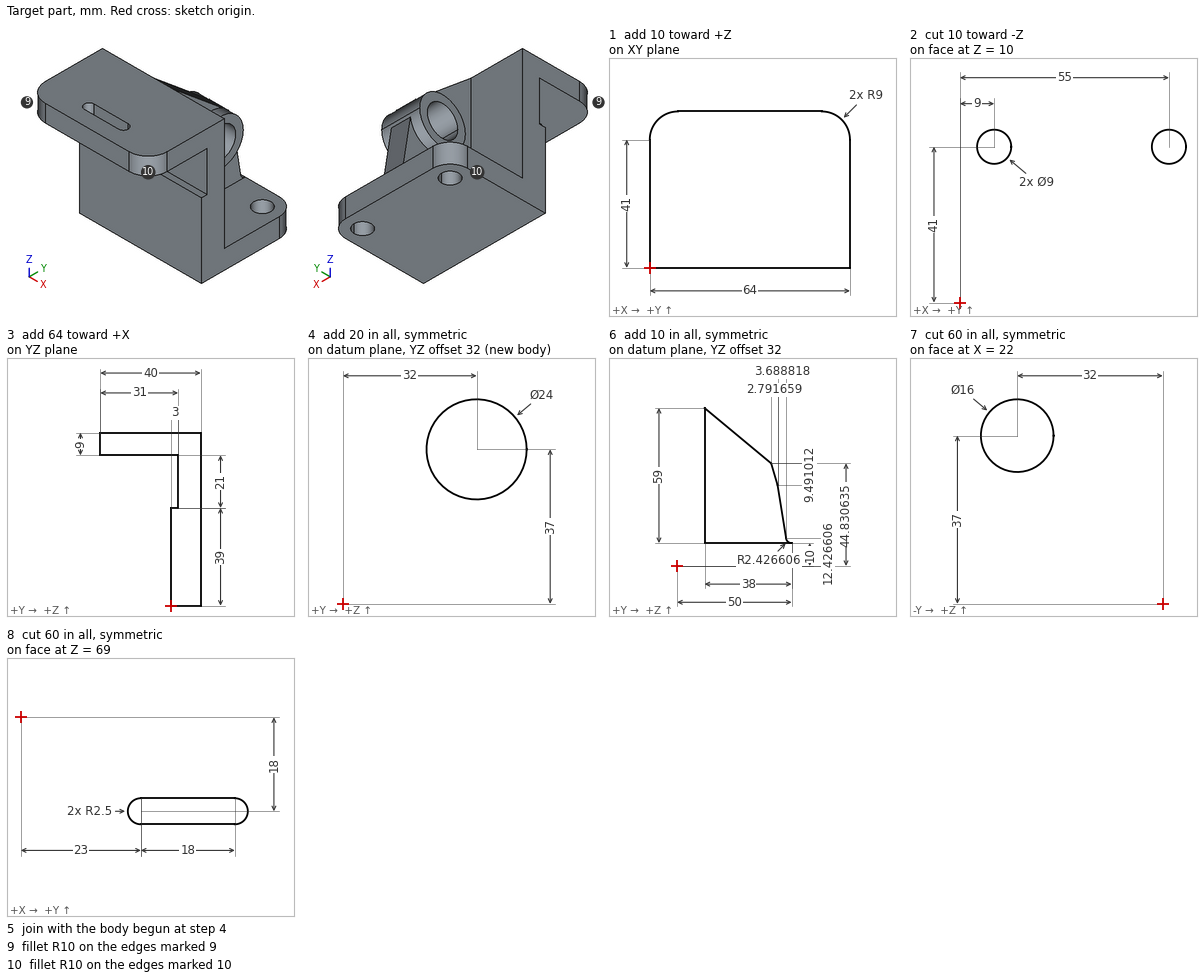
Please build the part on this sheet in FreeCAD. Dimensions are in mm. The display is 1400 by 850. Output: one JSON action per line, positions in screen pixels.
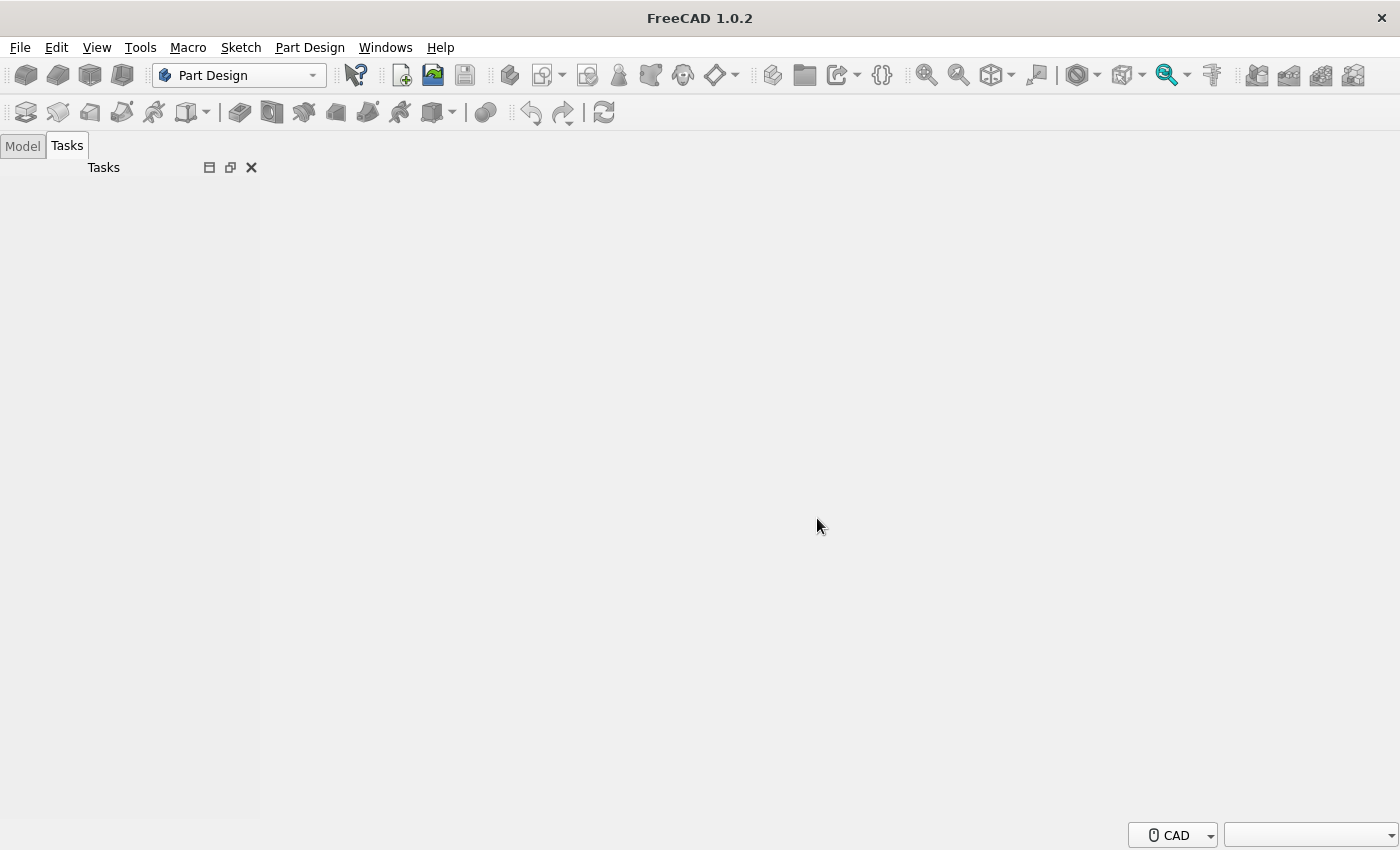
{"action": "left_click", "coordinate": [402, 76]}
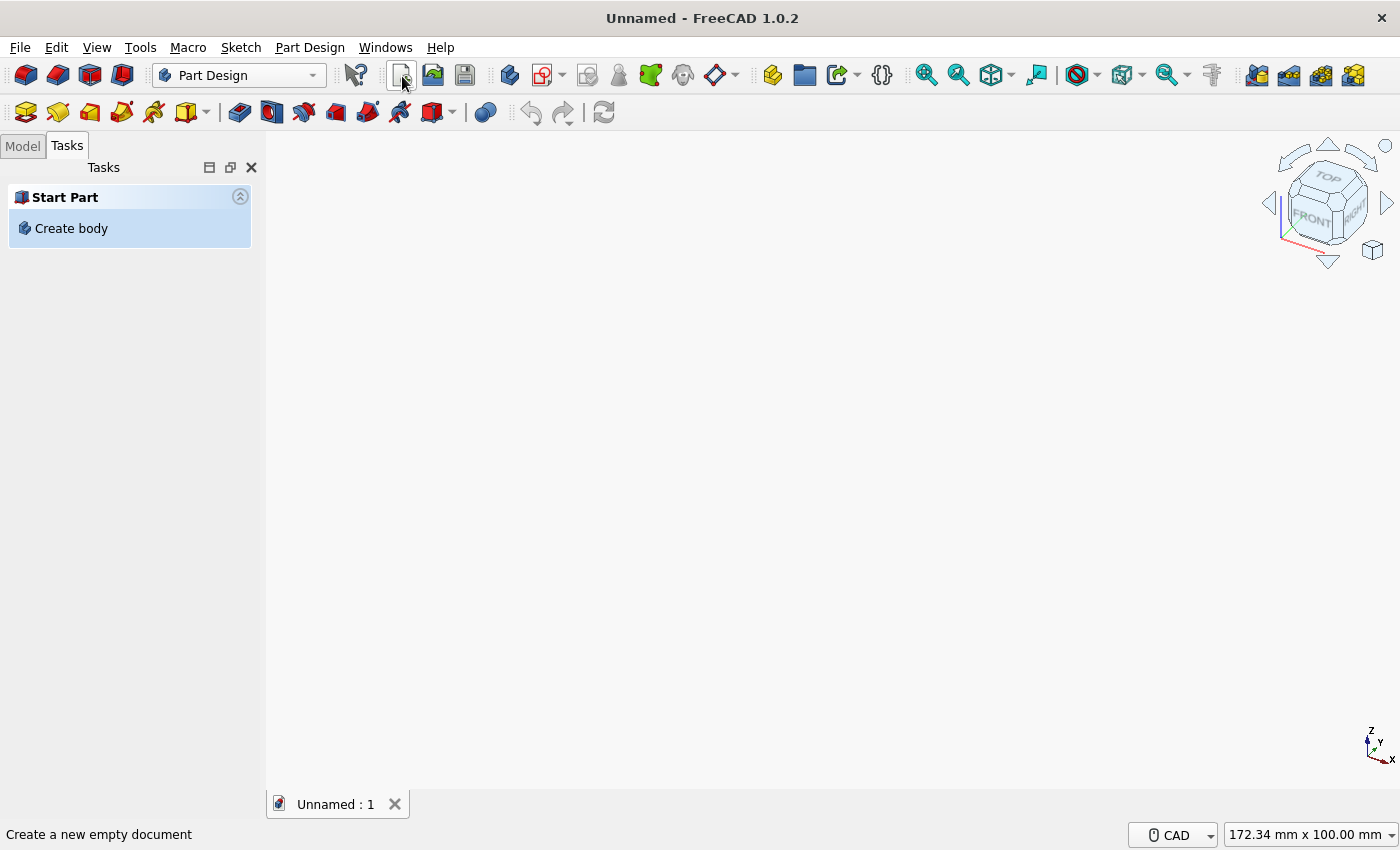
{"action": "left_click", "coordinate": [542, 76]}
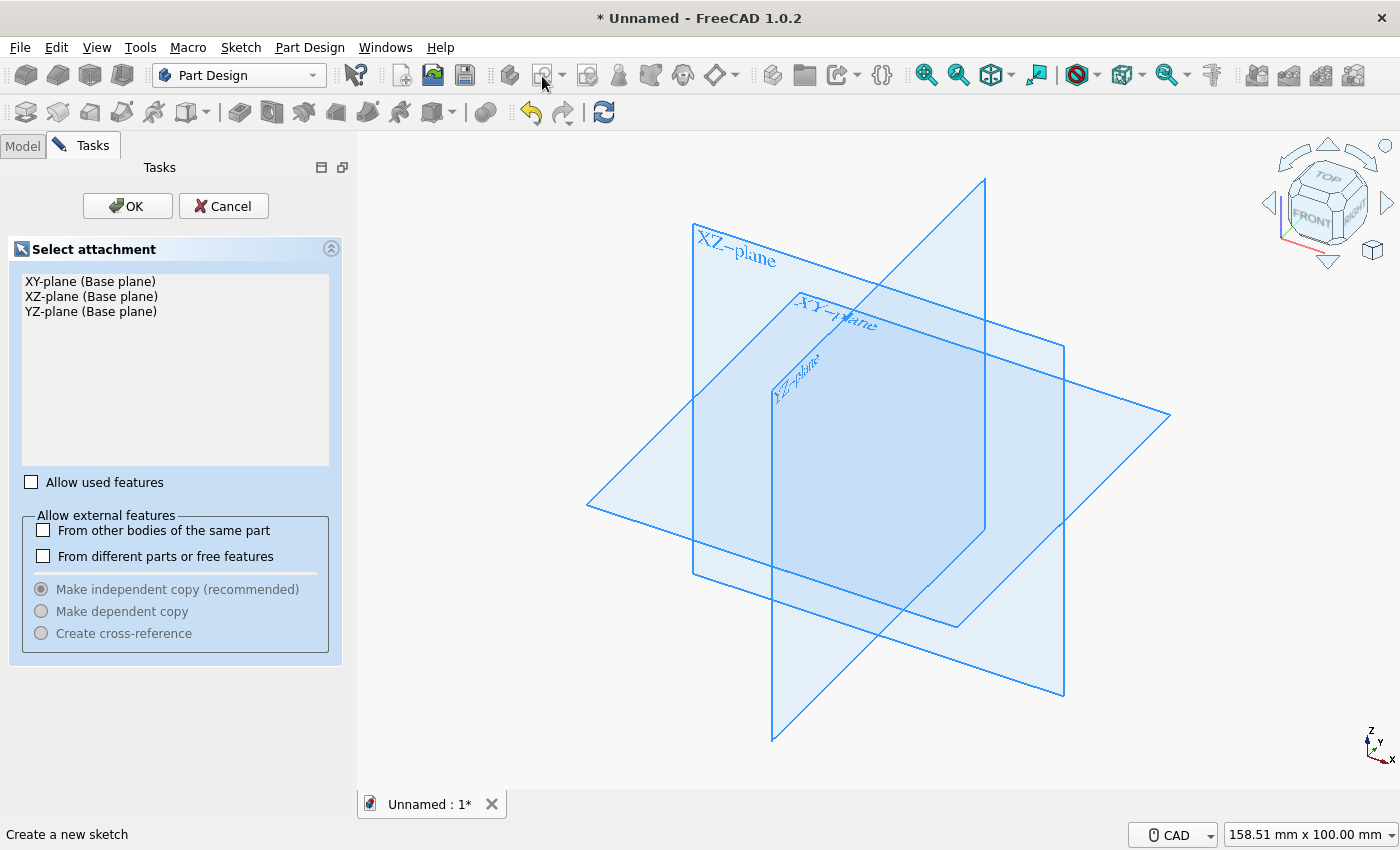
{"action": "left_click", "coordinate": [82, 282]}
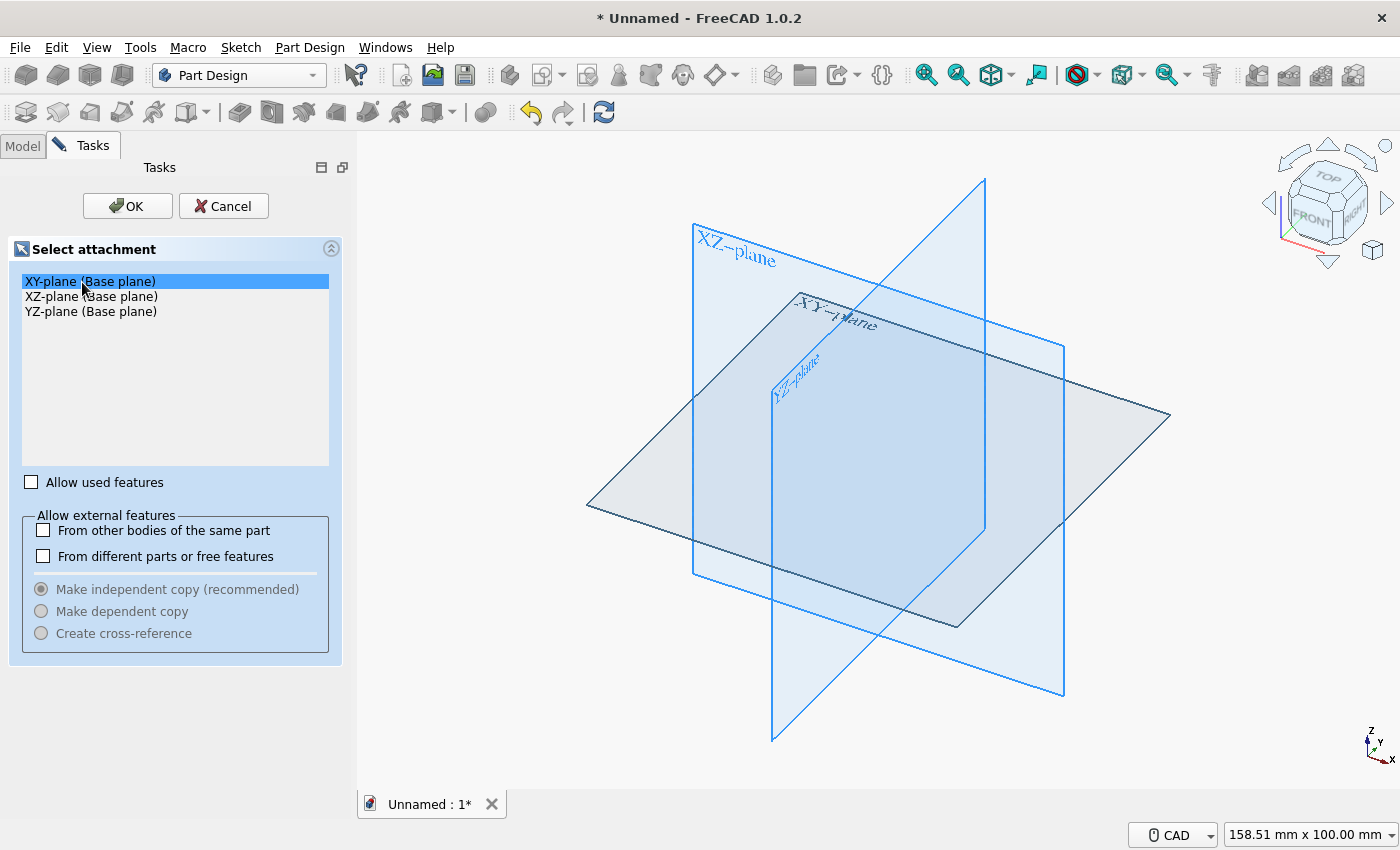
{"action": "left_click", "coordinate": [128, 206]}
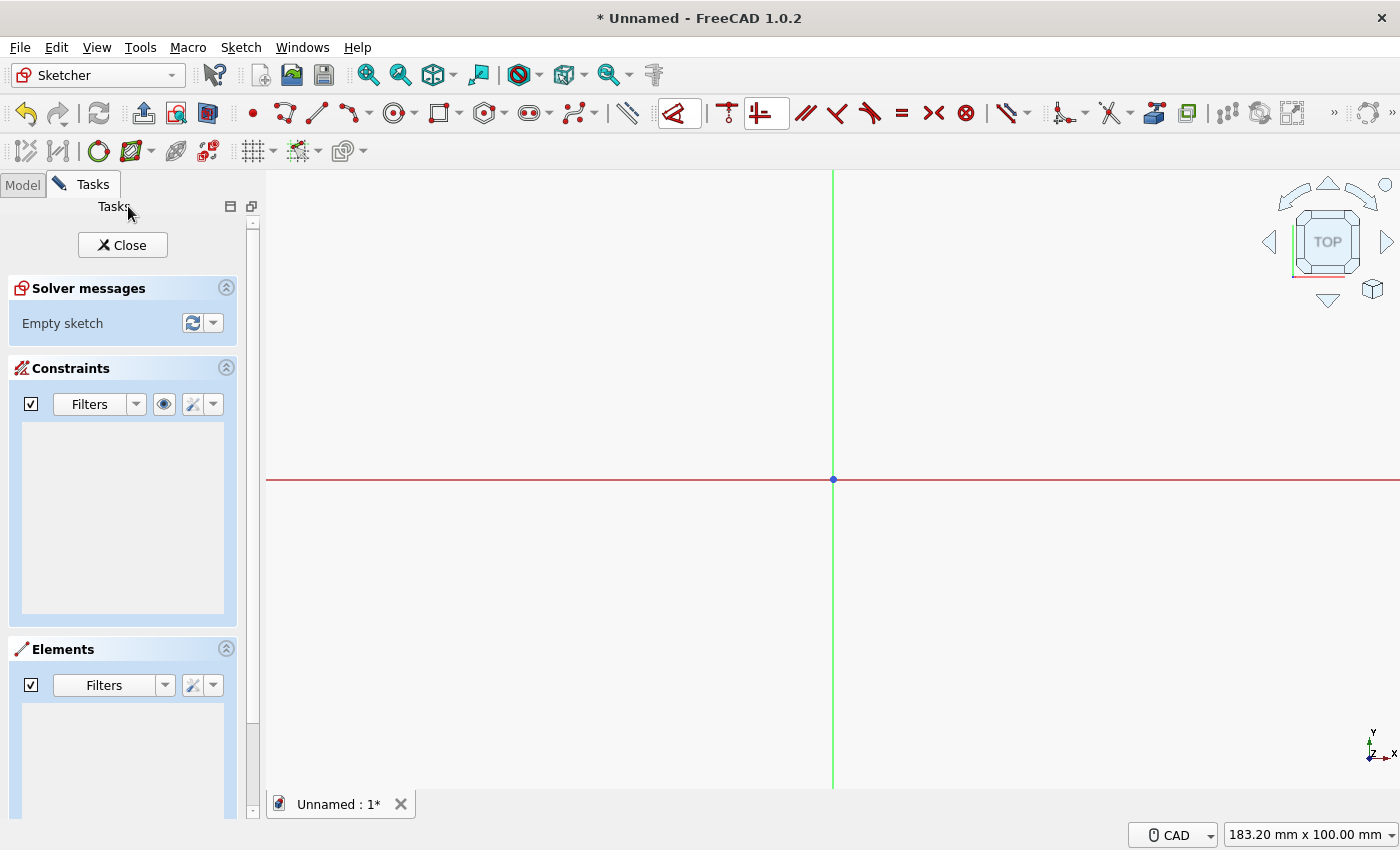
{"action": "scroll", "coordinate": [294, 761], "scroll_direction": "down", "scroll_amount": 1}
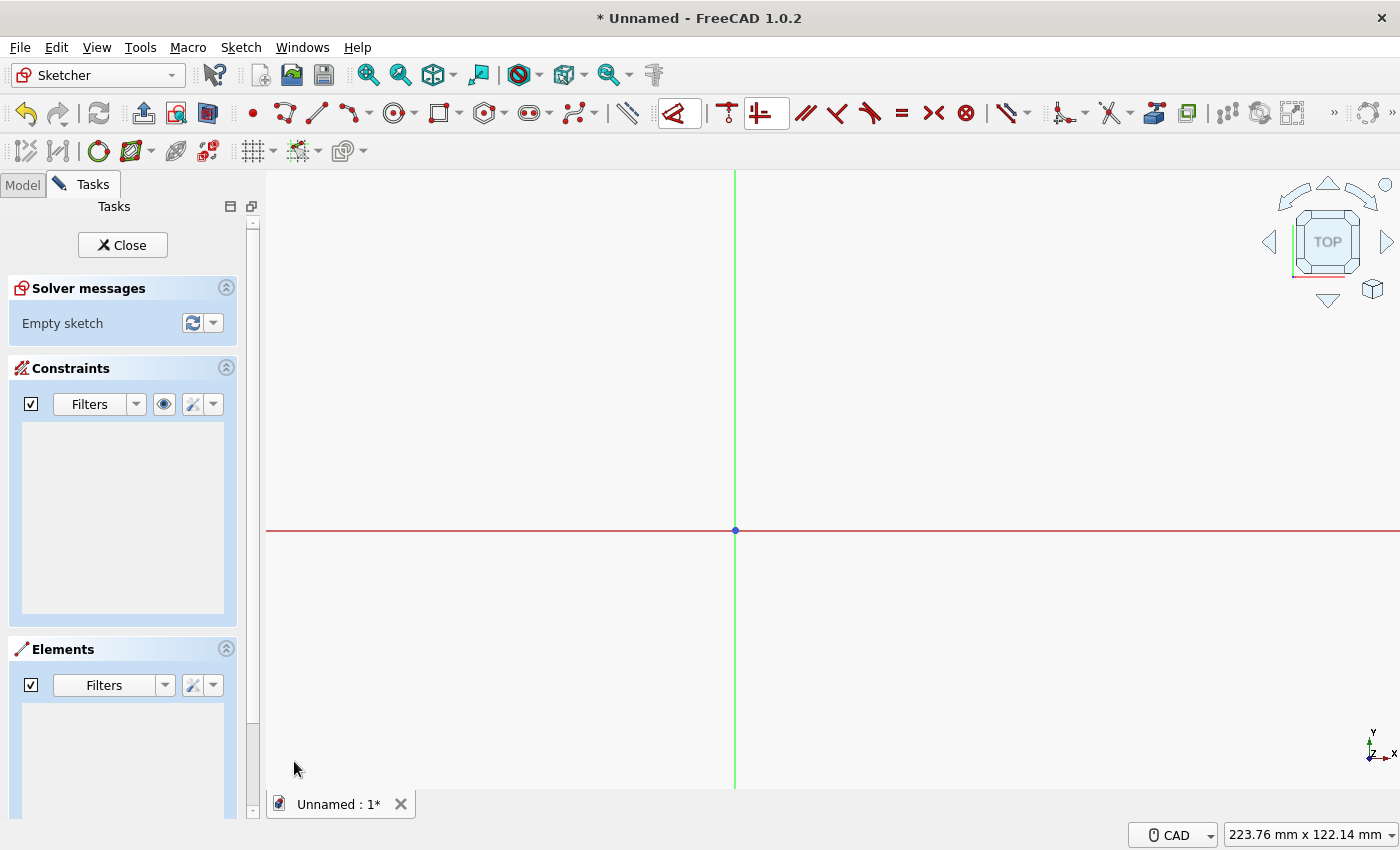
{"action": "scroll", "coordinate": [1168, 250], "scroll_direction": "up", "scroll_amount": 2}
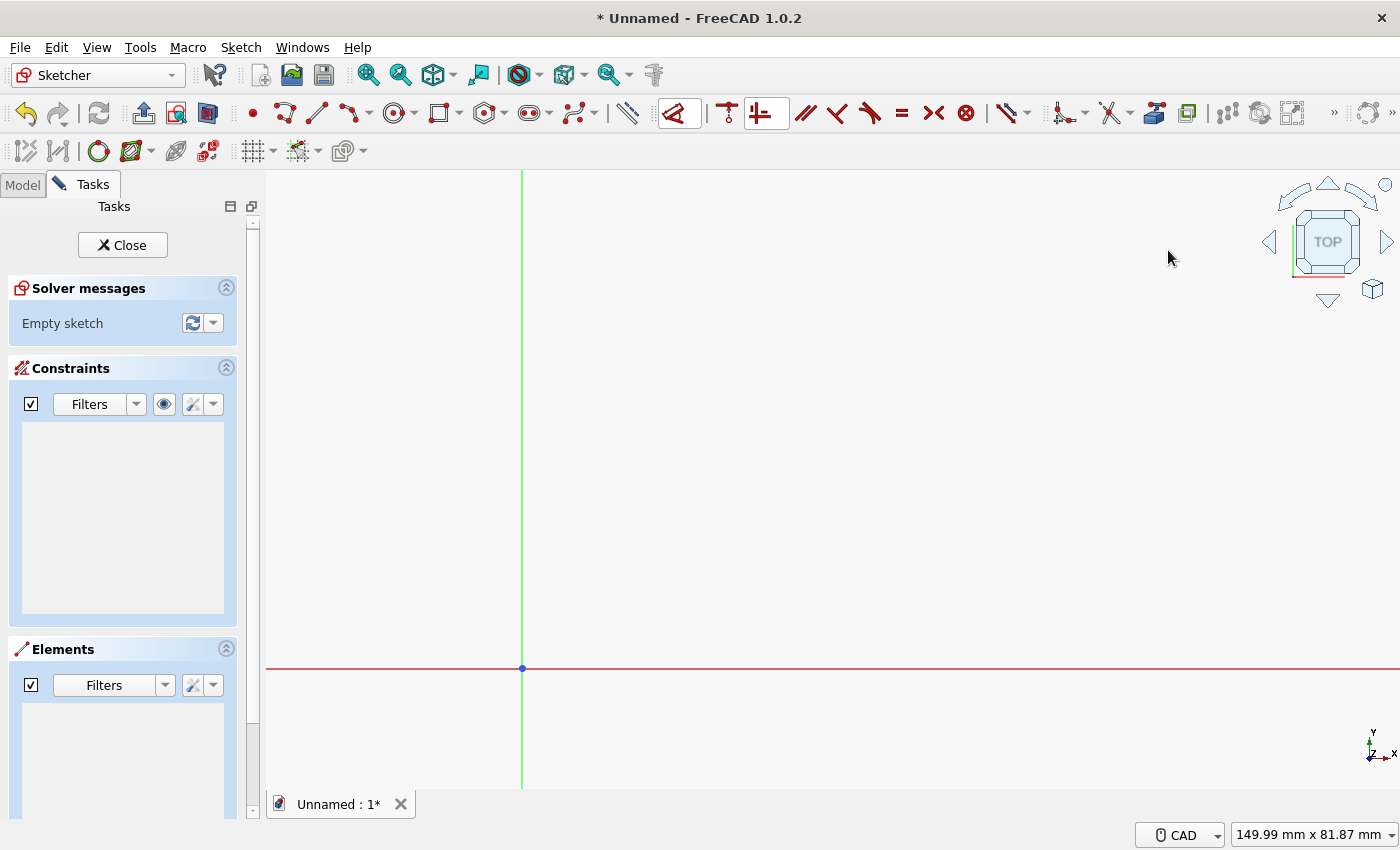
{"action": "left_click", "coordinate": [286, 114]}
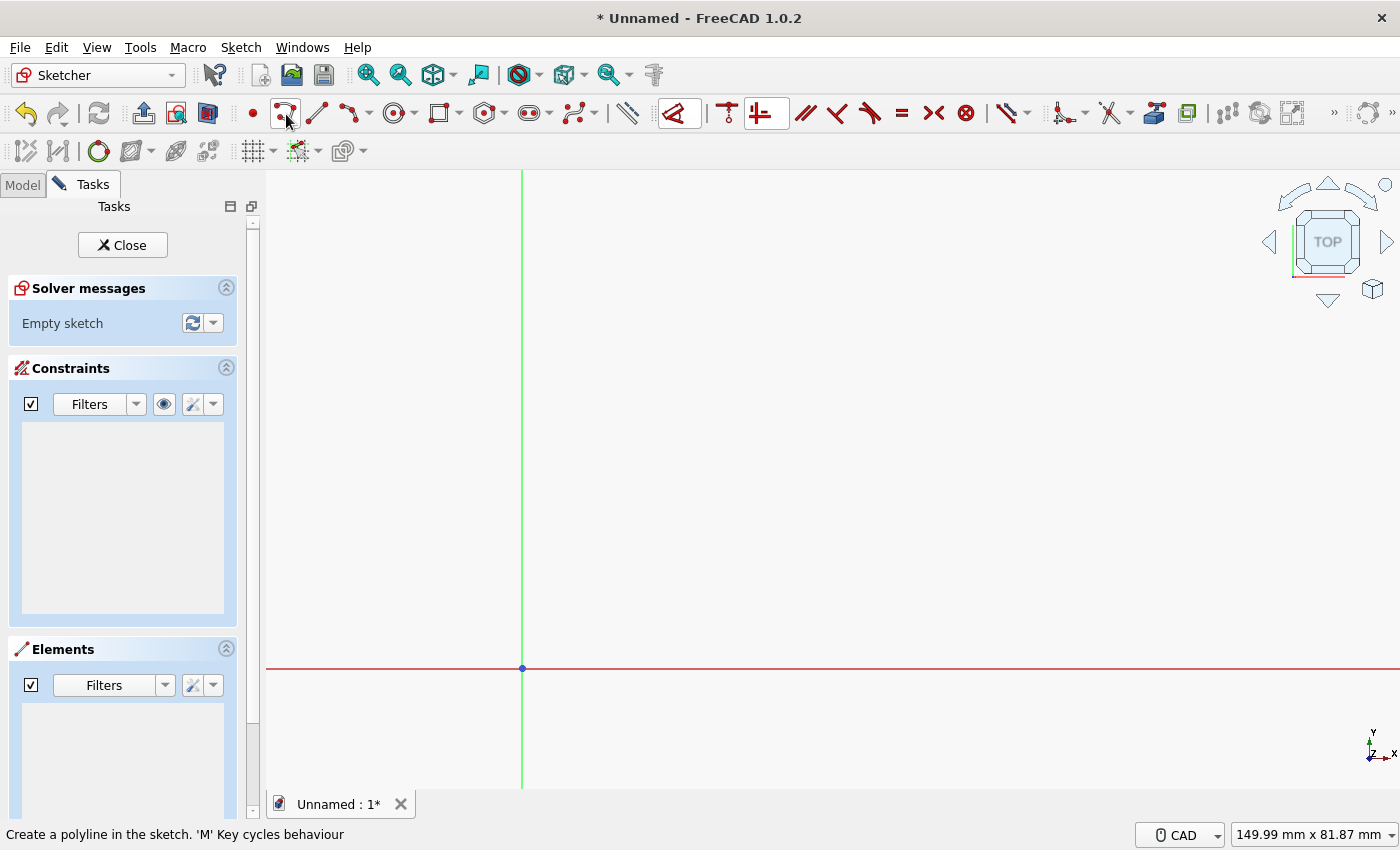
{"action": "left_click", "coordinate": [522, 359]}
{"action": "left_click", "coordinate": [522, 669]}
{"action": "left_click", "coordinate": [1006, 660]}
{"action": "left_click", "coordinate": [1006, 359]}
{"action": "right_click", "coordinate": [1006, 359]}